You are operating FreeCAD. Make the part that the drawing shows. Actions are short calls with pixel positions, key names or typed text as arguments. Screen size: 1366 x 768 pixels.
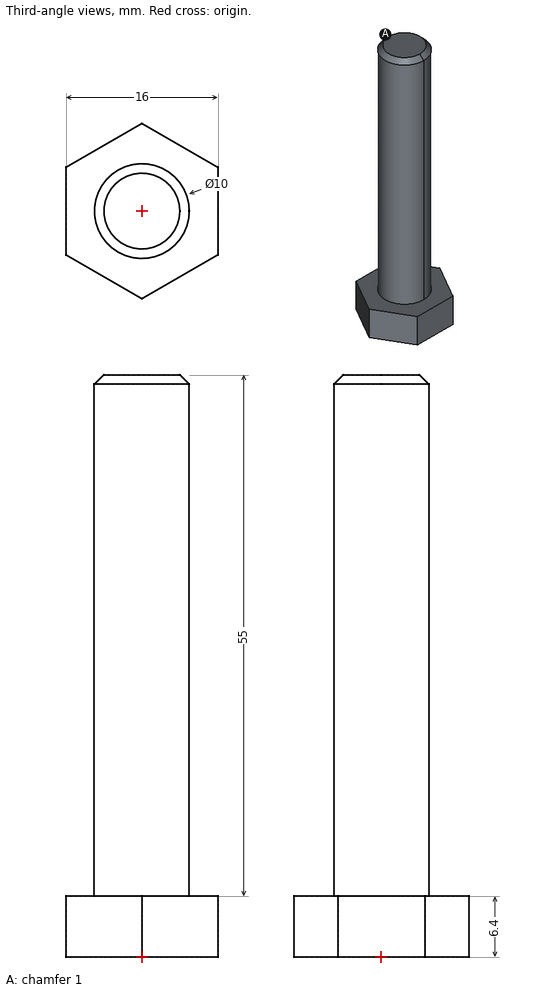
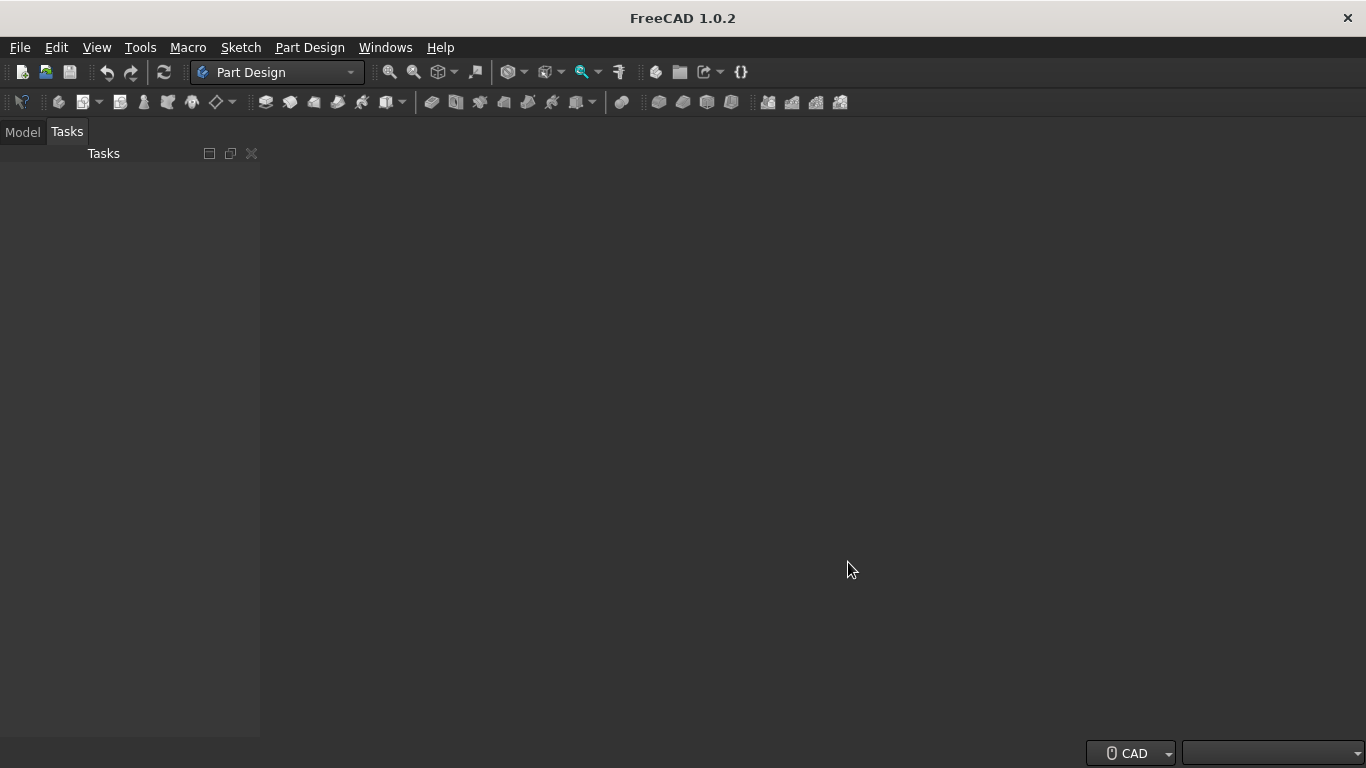
click(22, 72)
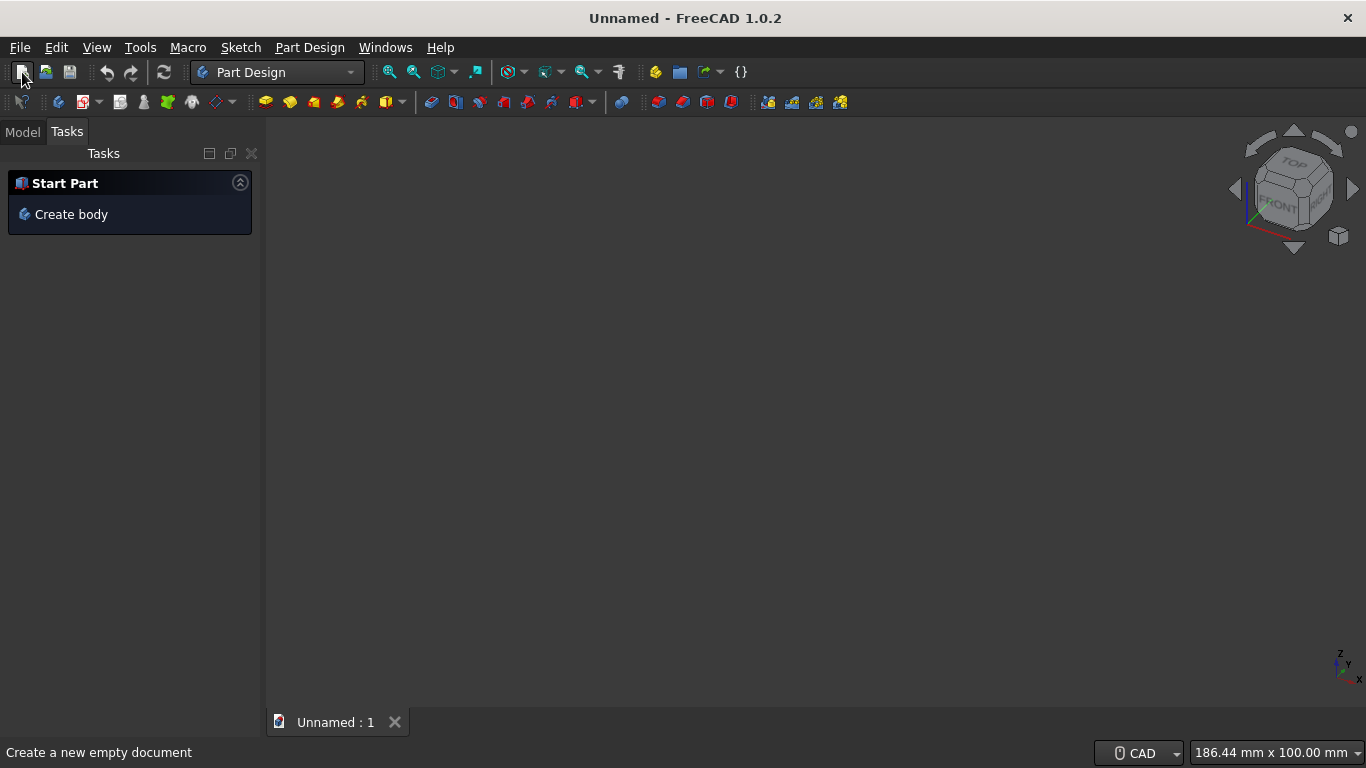
click(84, 102)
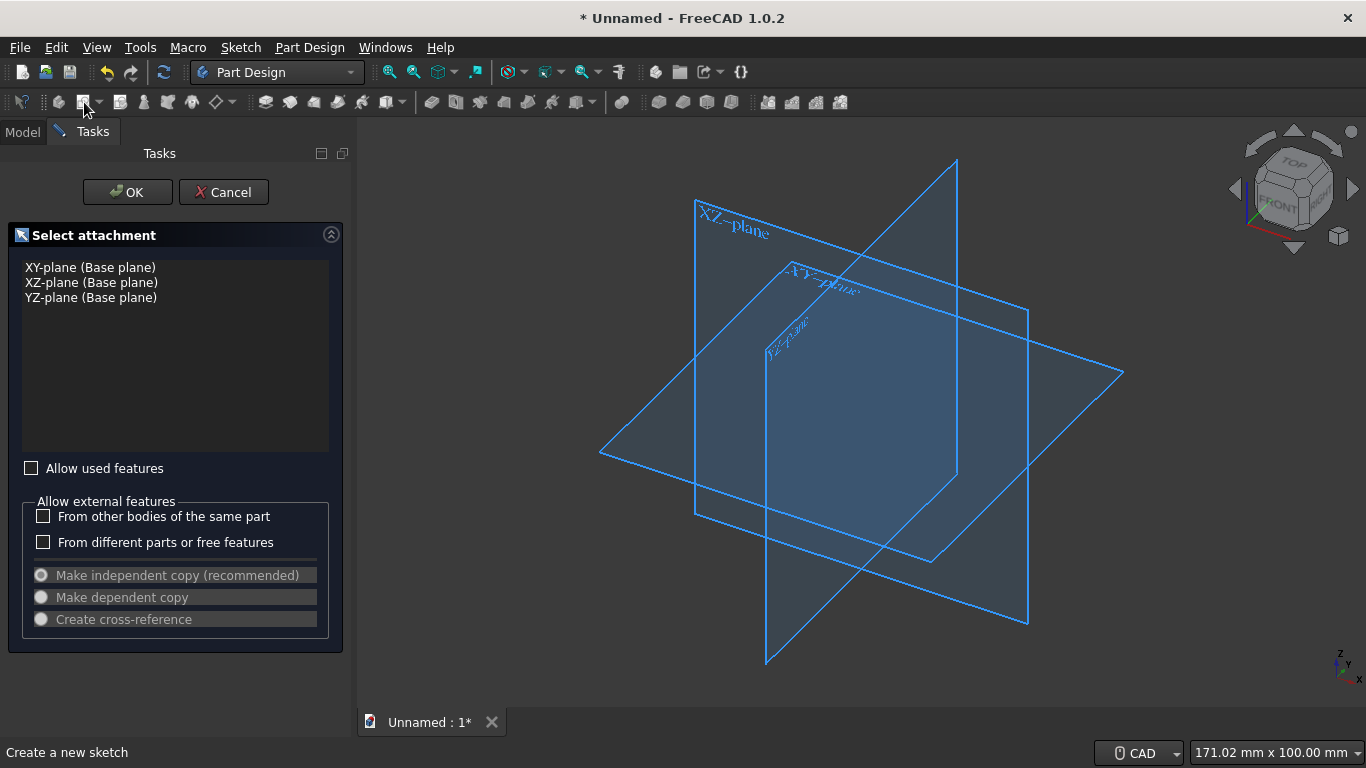
click(82, 268)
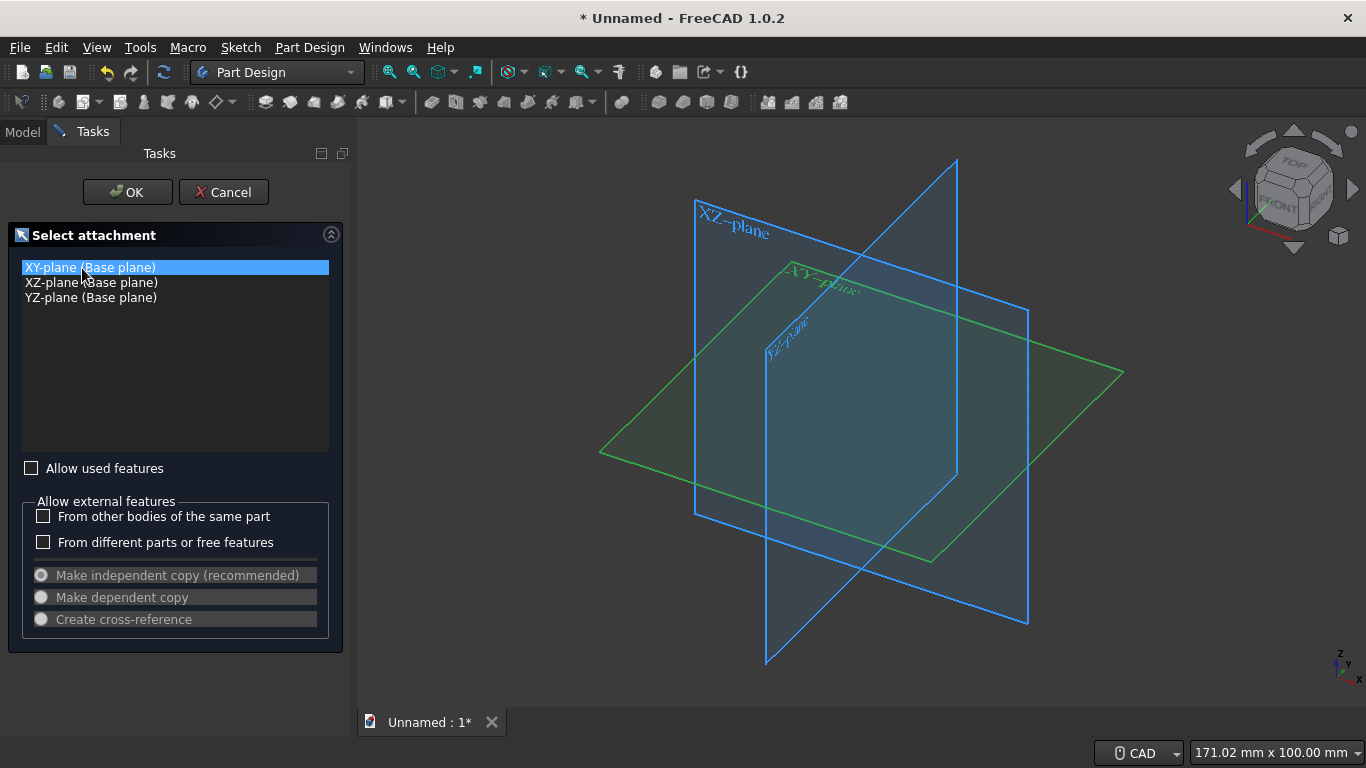
click(128, 192)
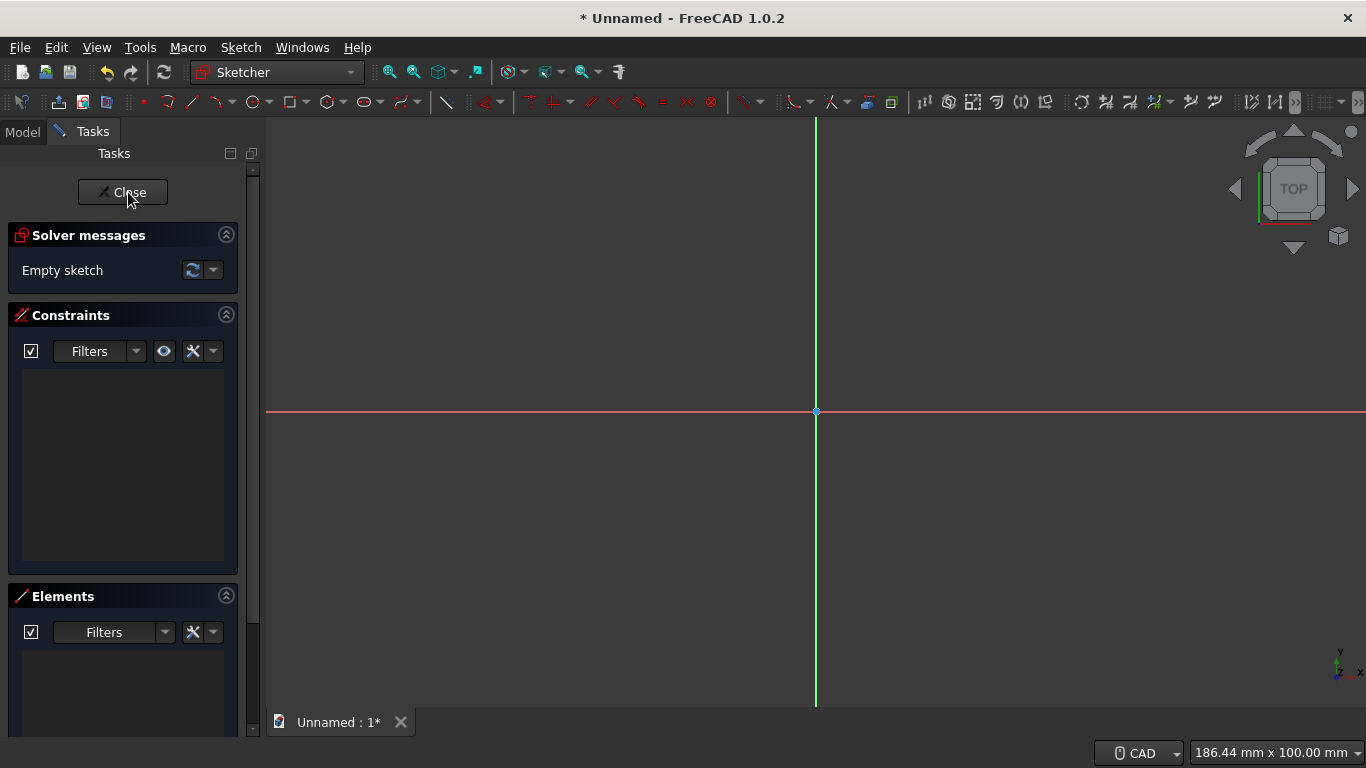
scroll(846, 412, up, 6)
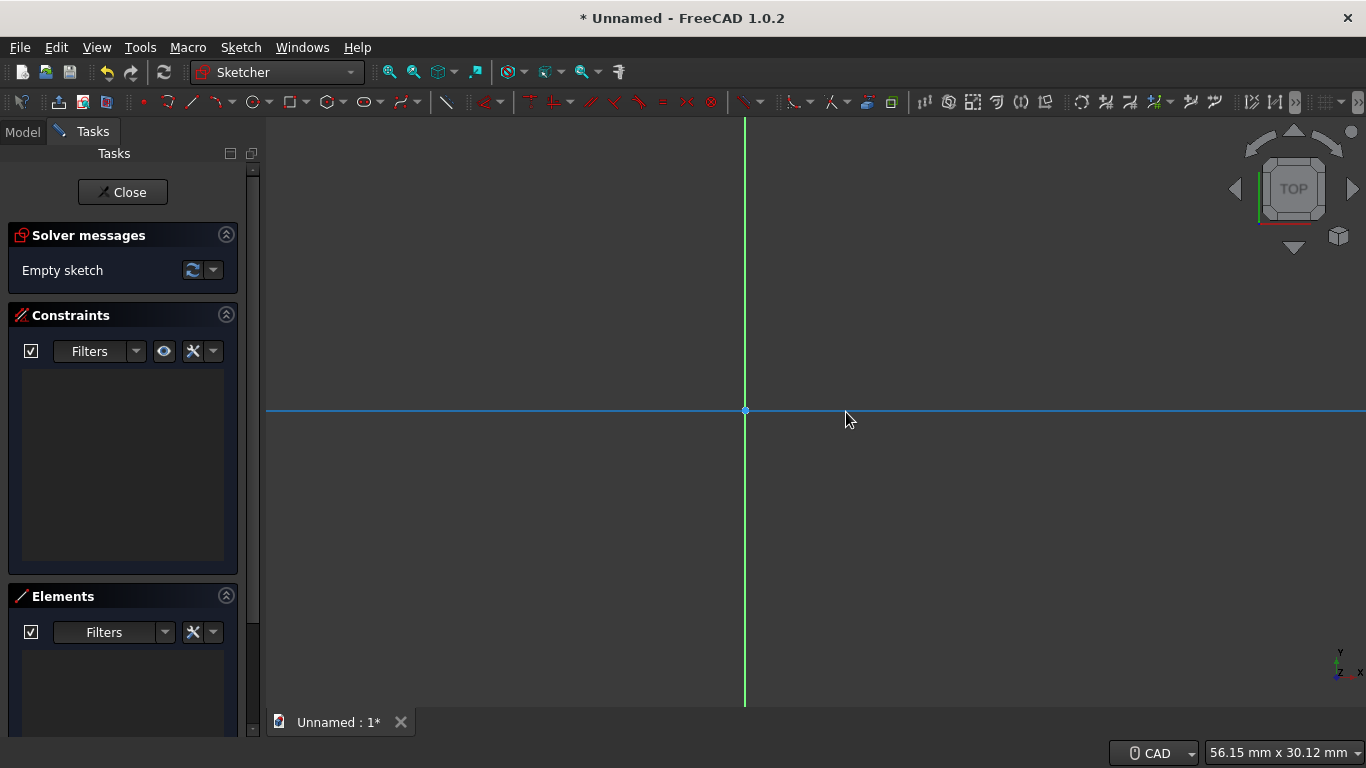
click(328, 102)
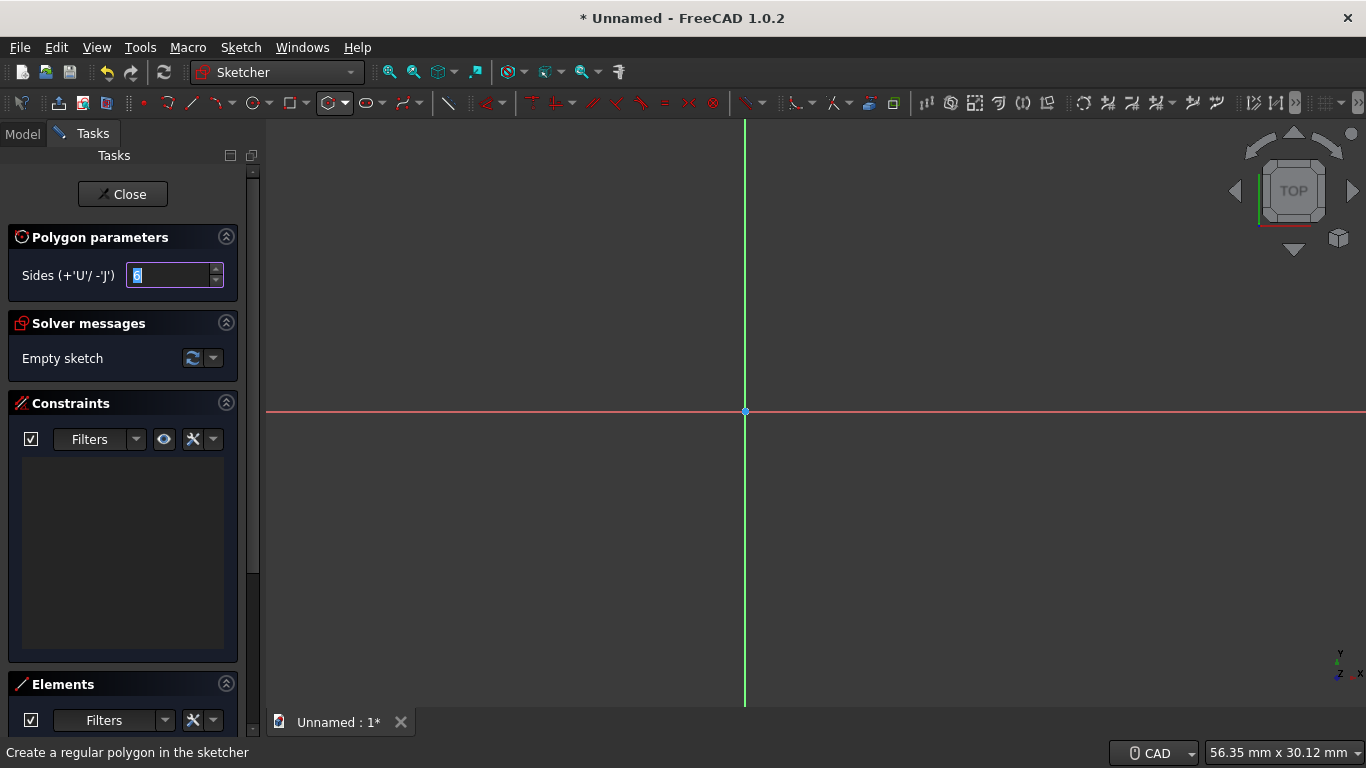
click(745, 412)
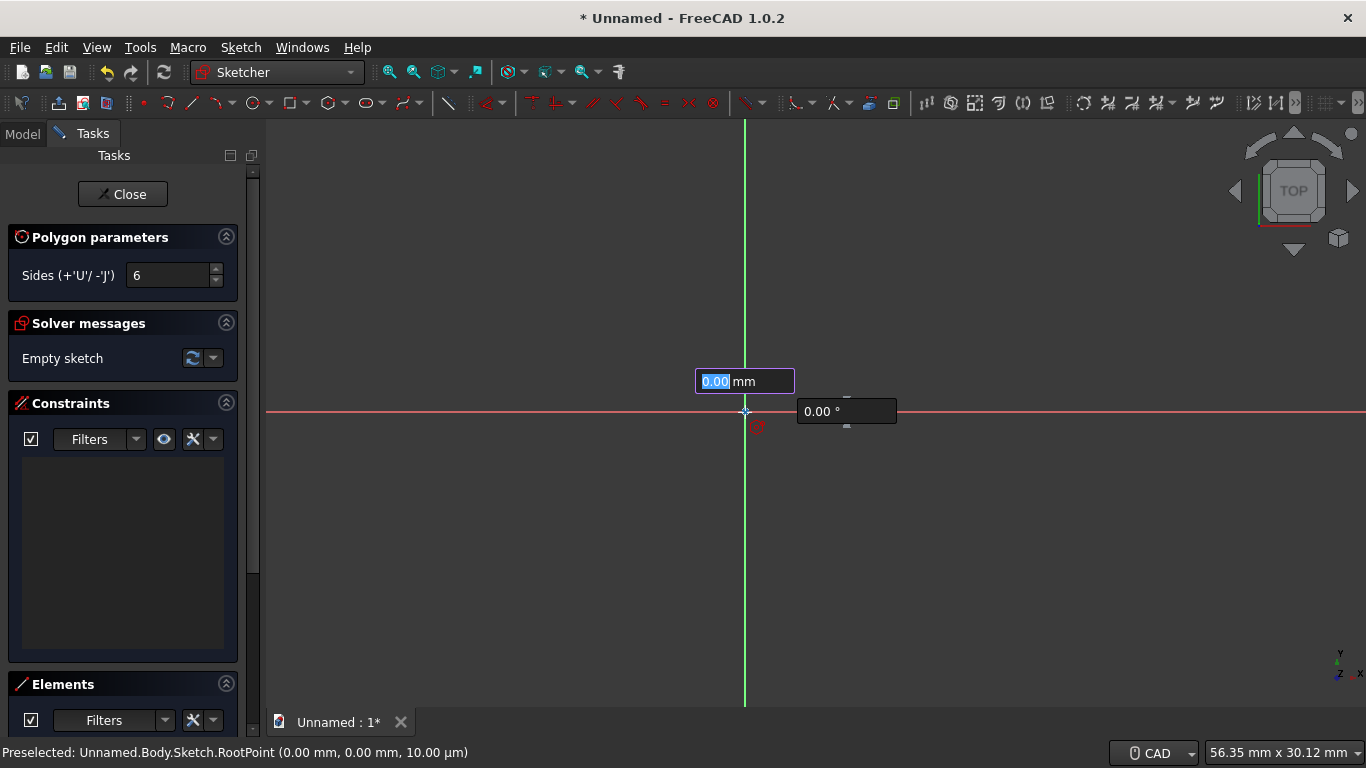
click(745, 232)
right_click(745, 232)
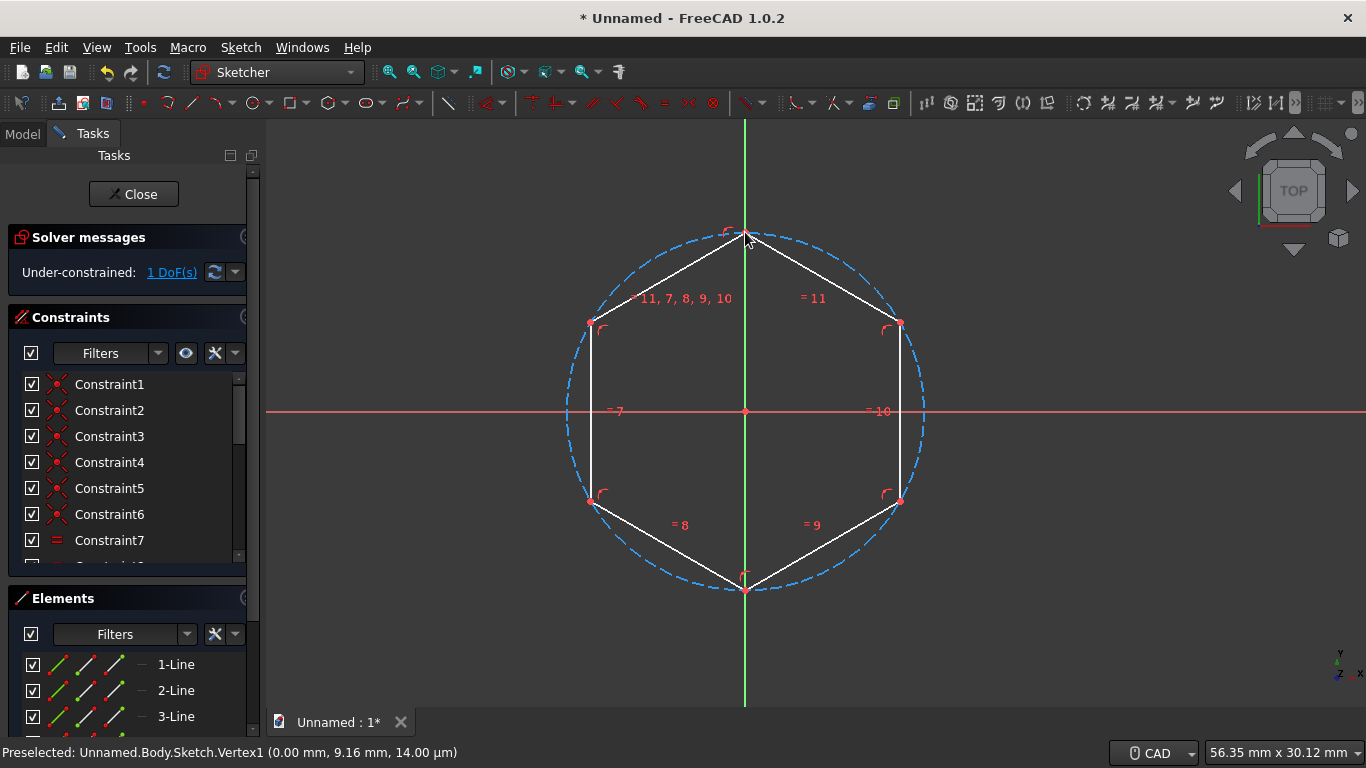
click(486, 104)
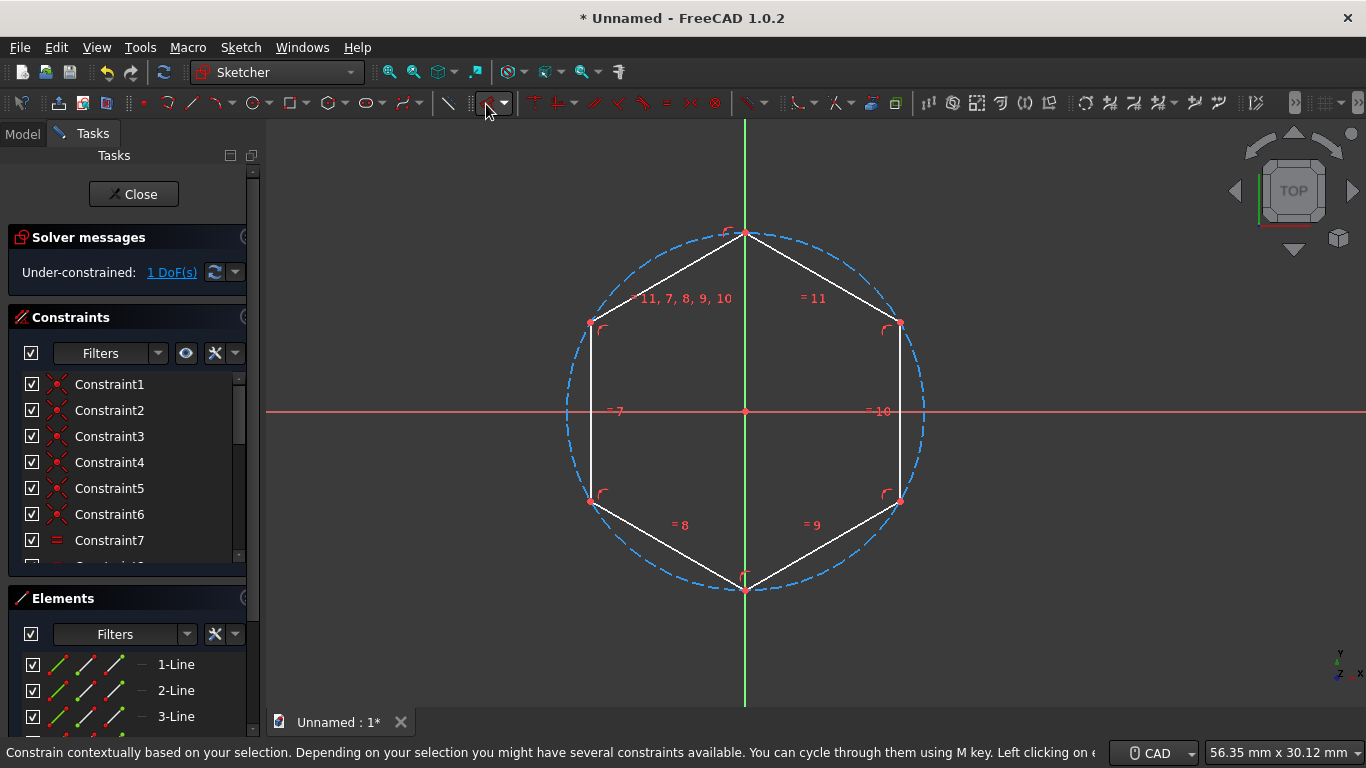
click(591, 322)